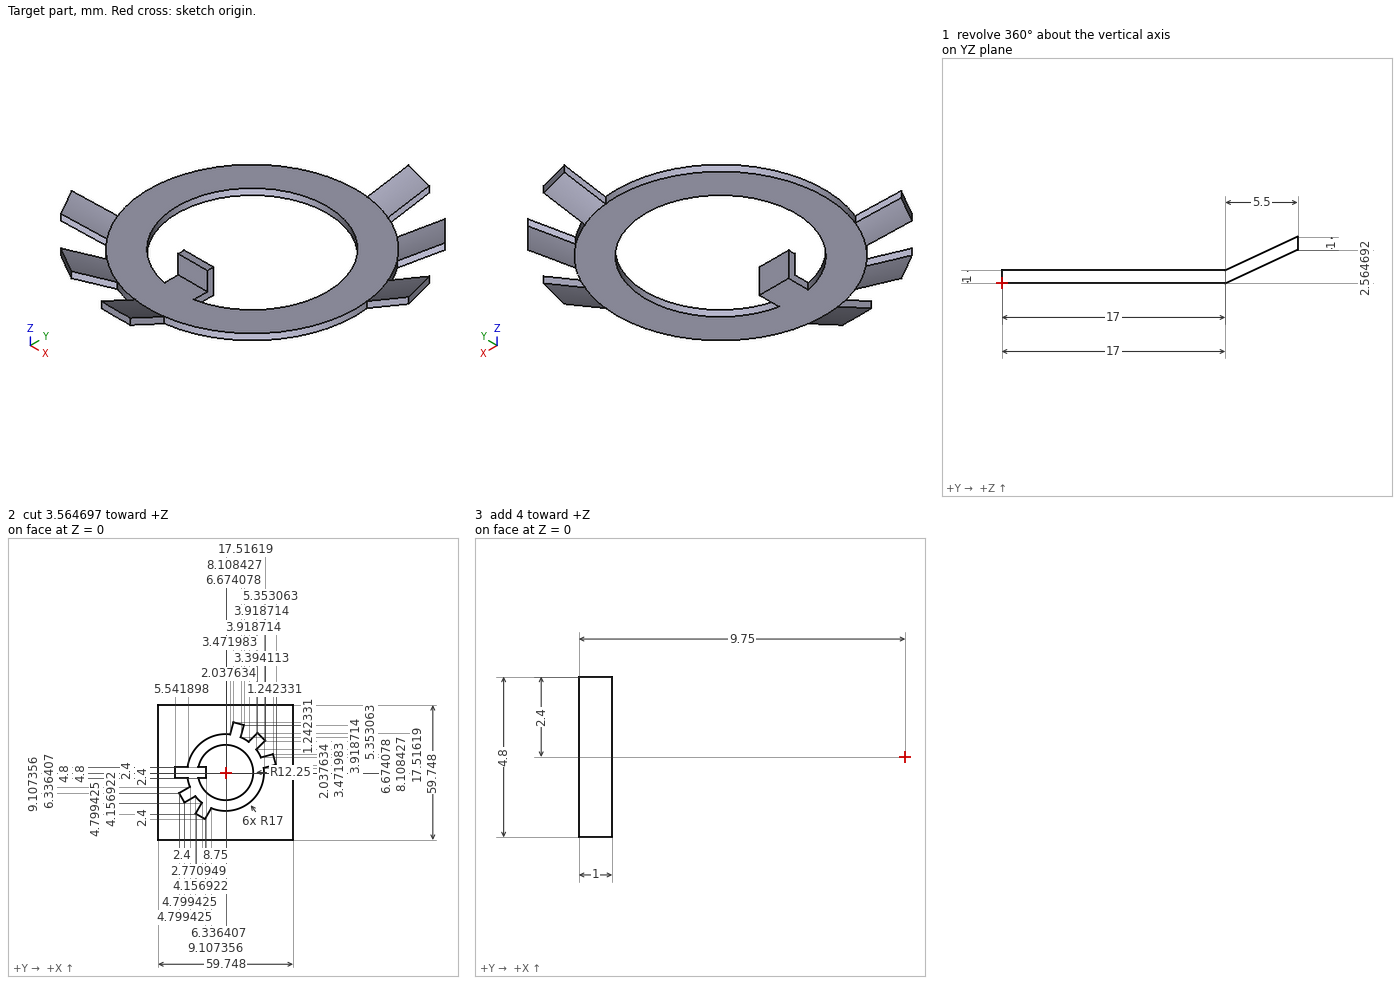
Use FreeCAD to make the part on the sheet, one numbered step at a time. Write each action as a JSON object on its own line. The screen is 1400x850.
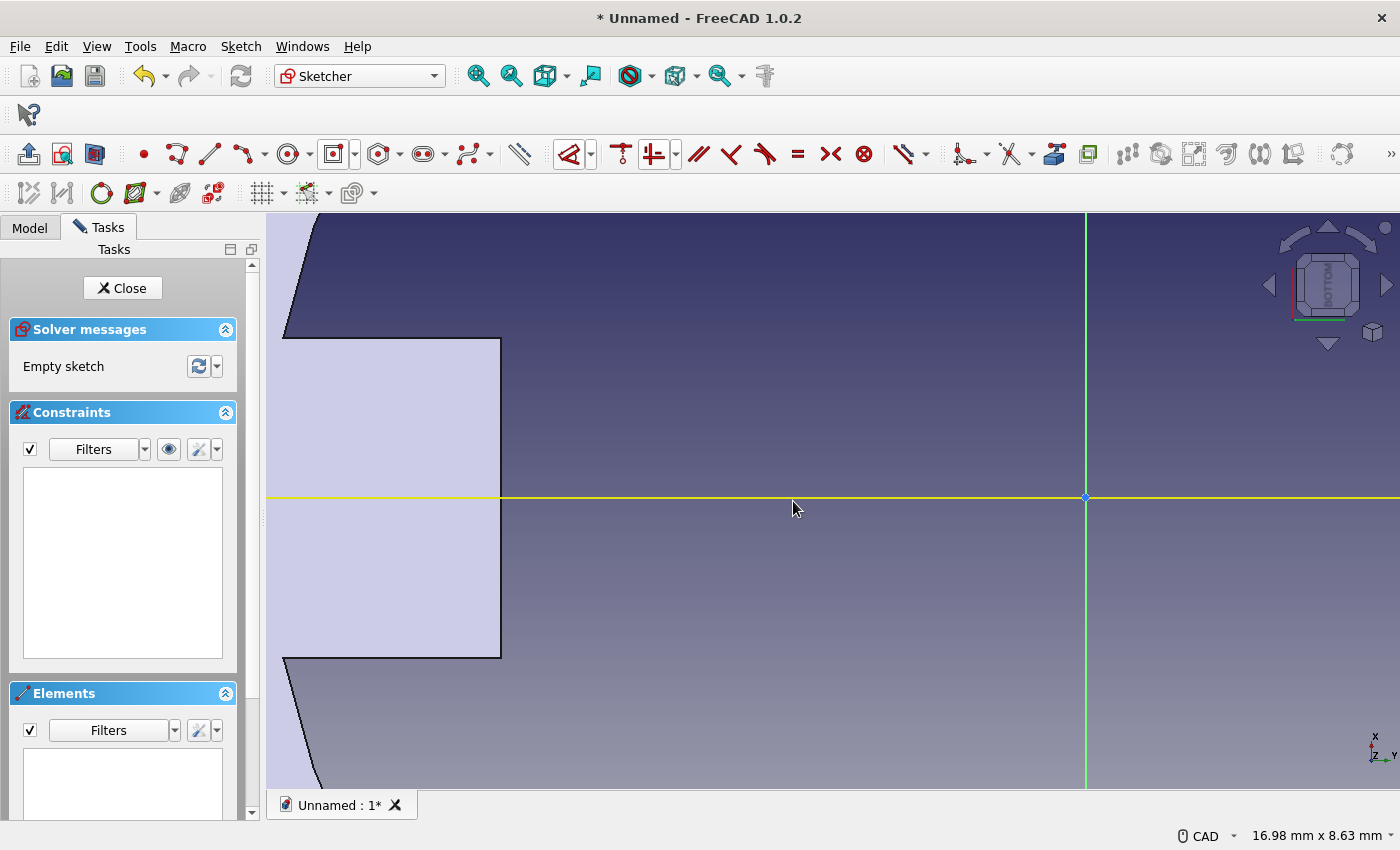
{"action": "left_click", "coordinate": [354, 154]}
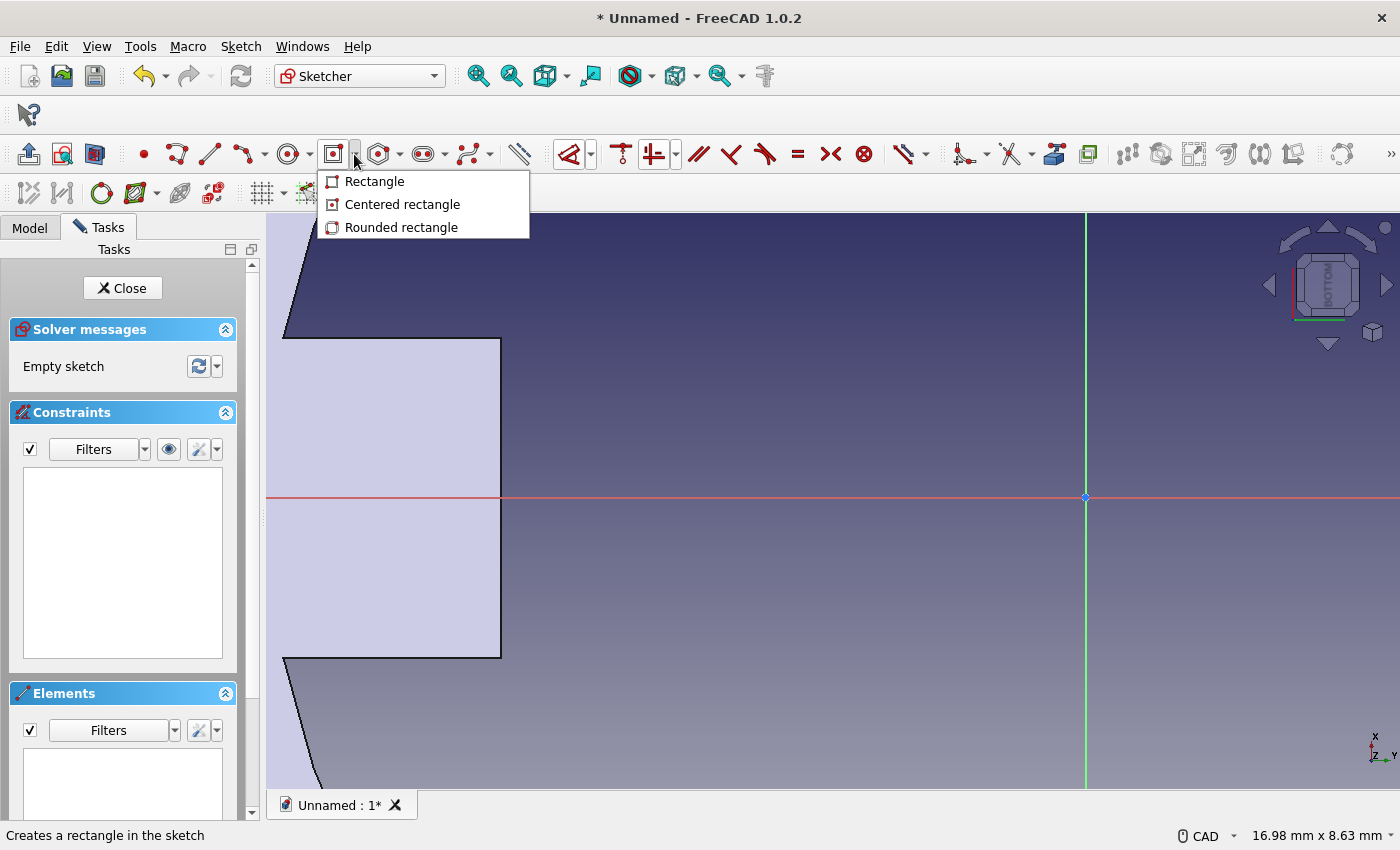
{"action": "left_click", "coordinate": [424, 182]}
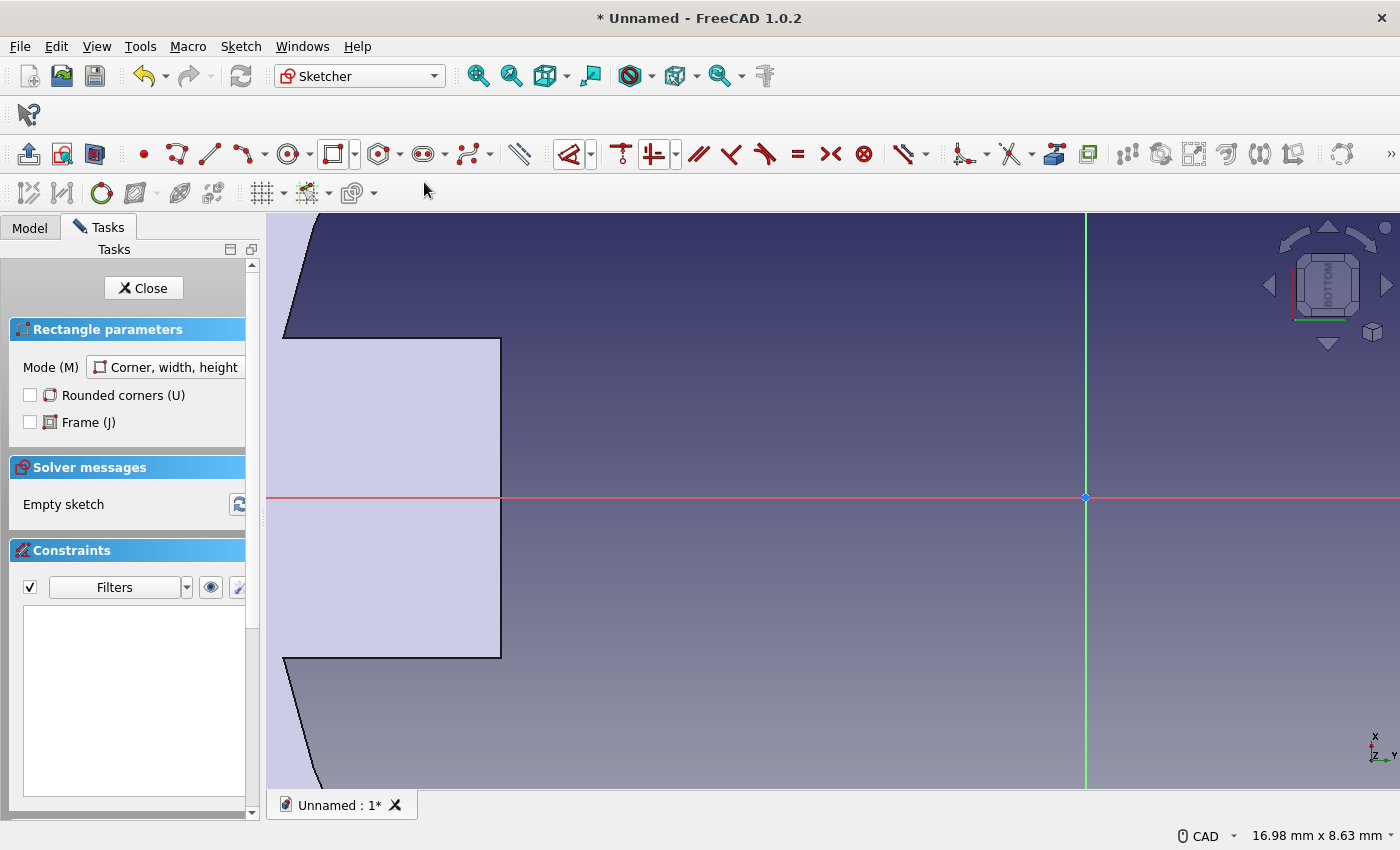
{"action": "left_click", "coordinate": [435, 338]}
{"action": "mouse_move", "coordinate": [501, 658]}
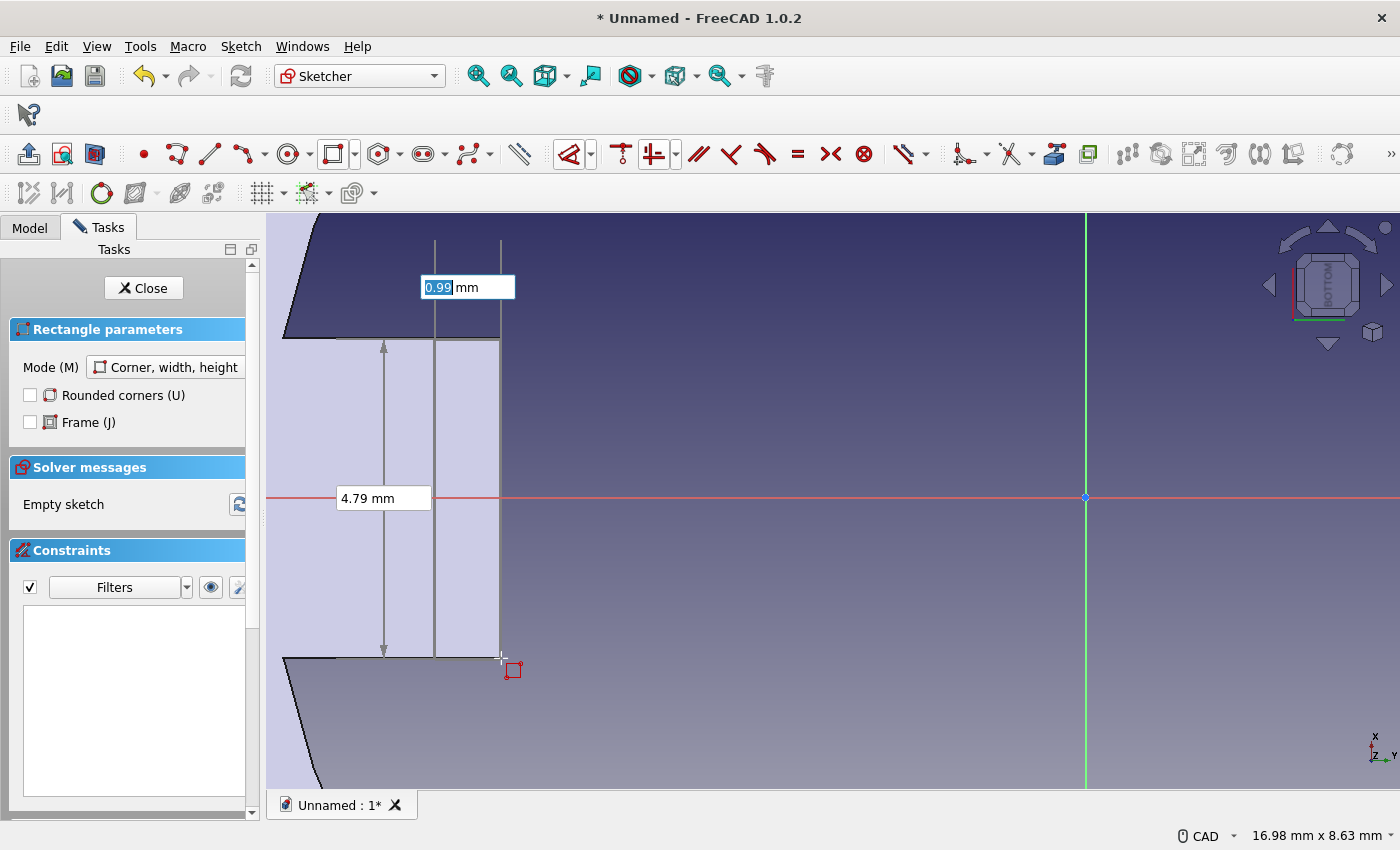
{"action": "type", "text": "1"}
{"action": "key", "text": "Tab"}
{"action": "type", "text": "4.8"}
{"action": "key", "text": "Return"}
{"action": "key", "text": "Escape"}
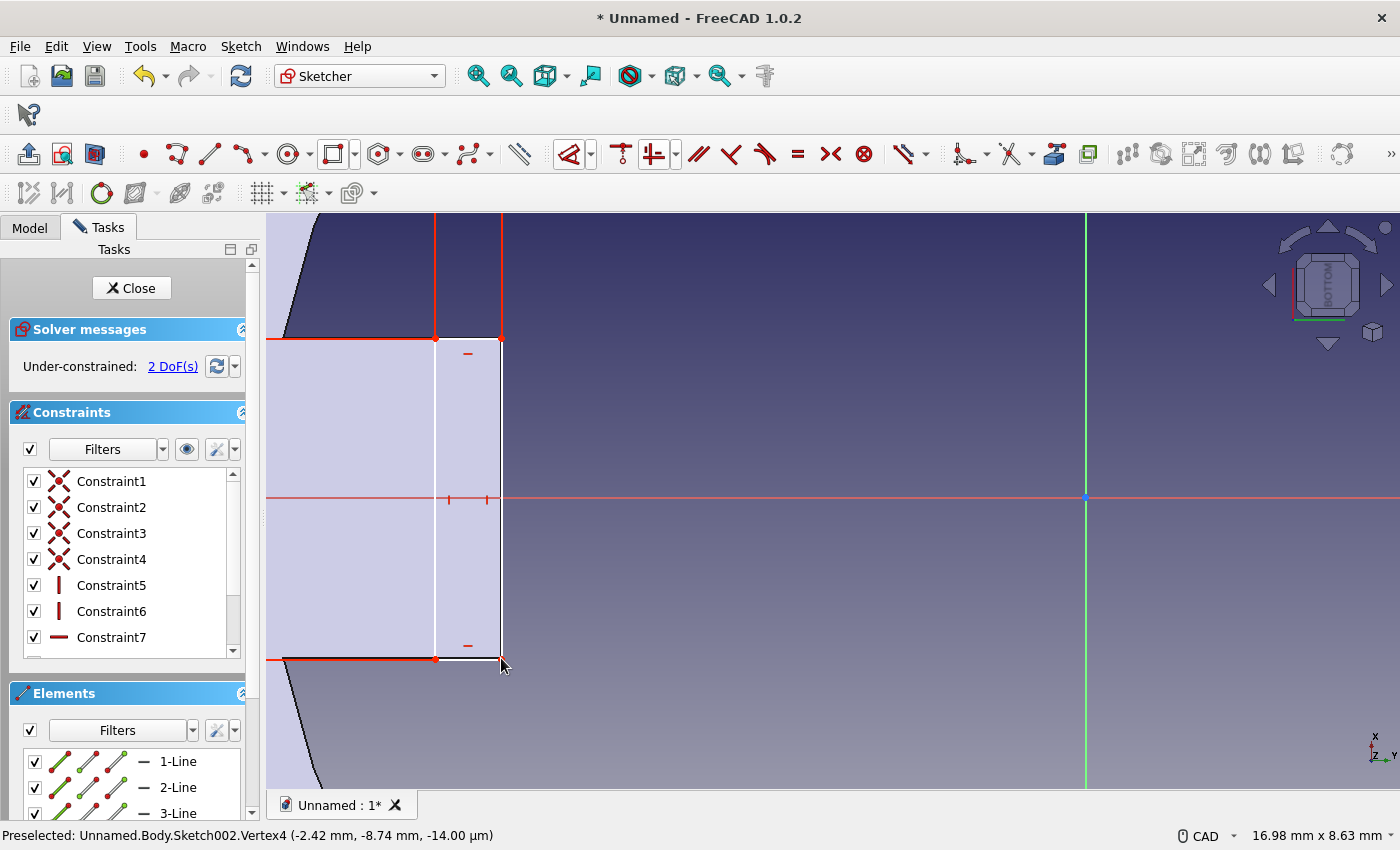
{"action": "left_click", "coordinate": [435, 339]}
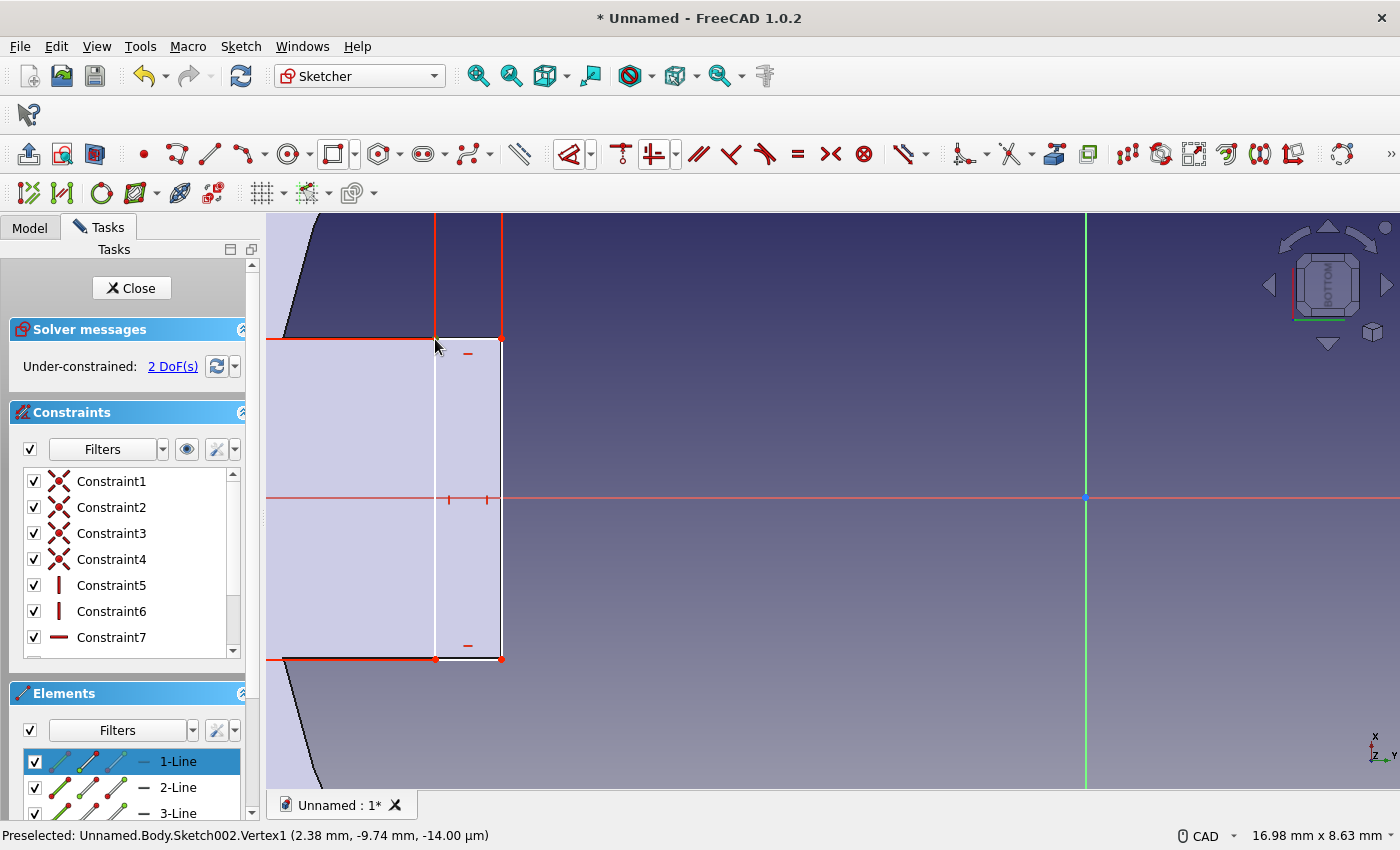
{"action": "left_click", "coordinate": [590, 154]}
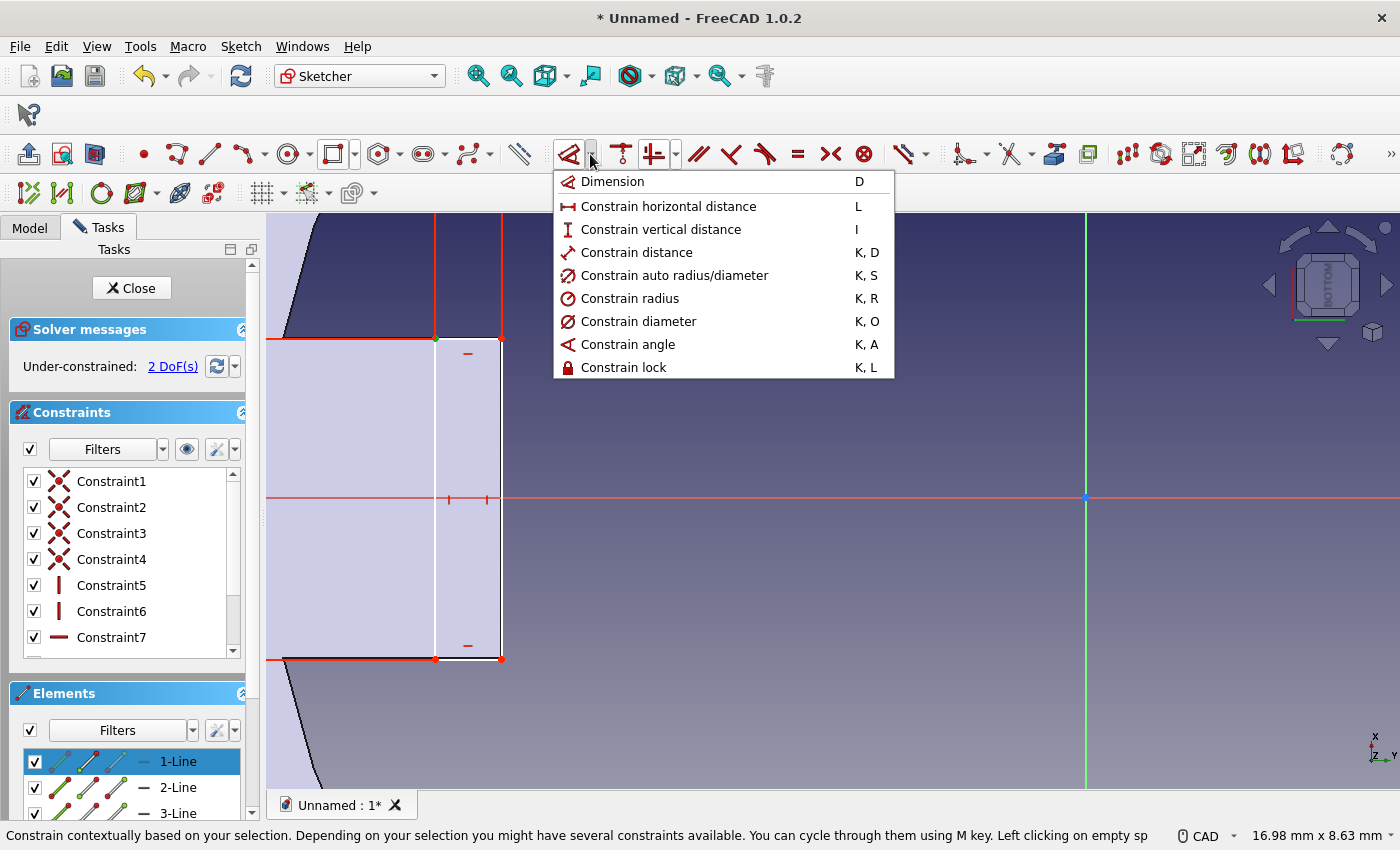
{"action": "left_click", "coordinate": [724, 230]}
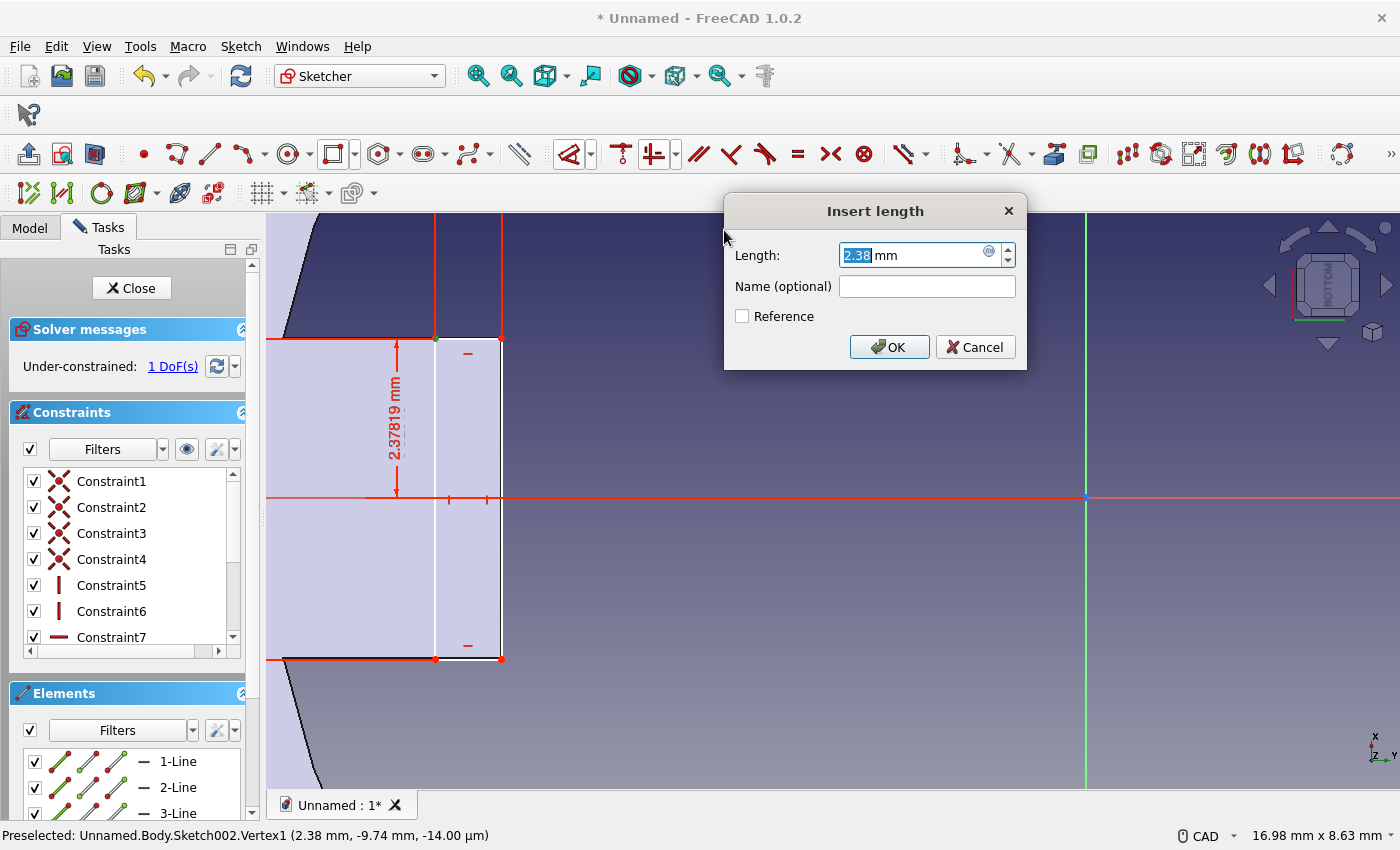
{"action": "type", "text": "2.4"}
{"action": "key", "text": "Return"}